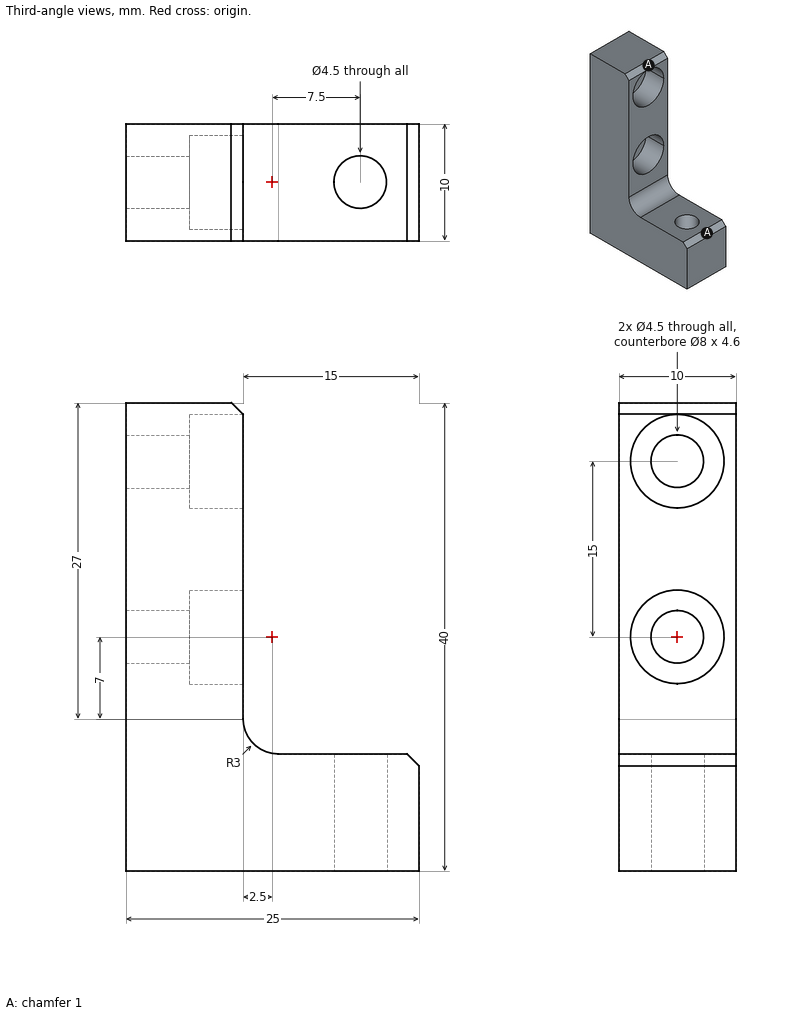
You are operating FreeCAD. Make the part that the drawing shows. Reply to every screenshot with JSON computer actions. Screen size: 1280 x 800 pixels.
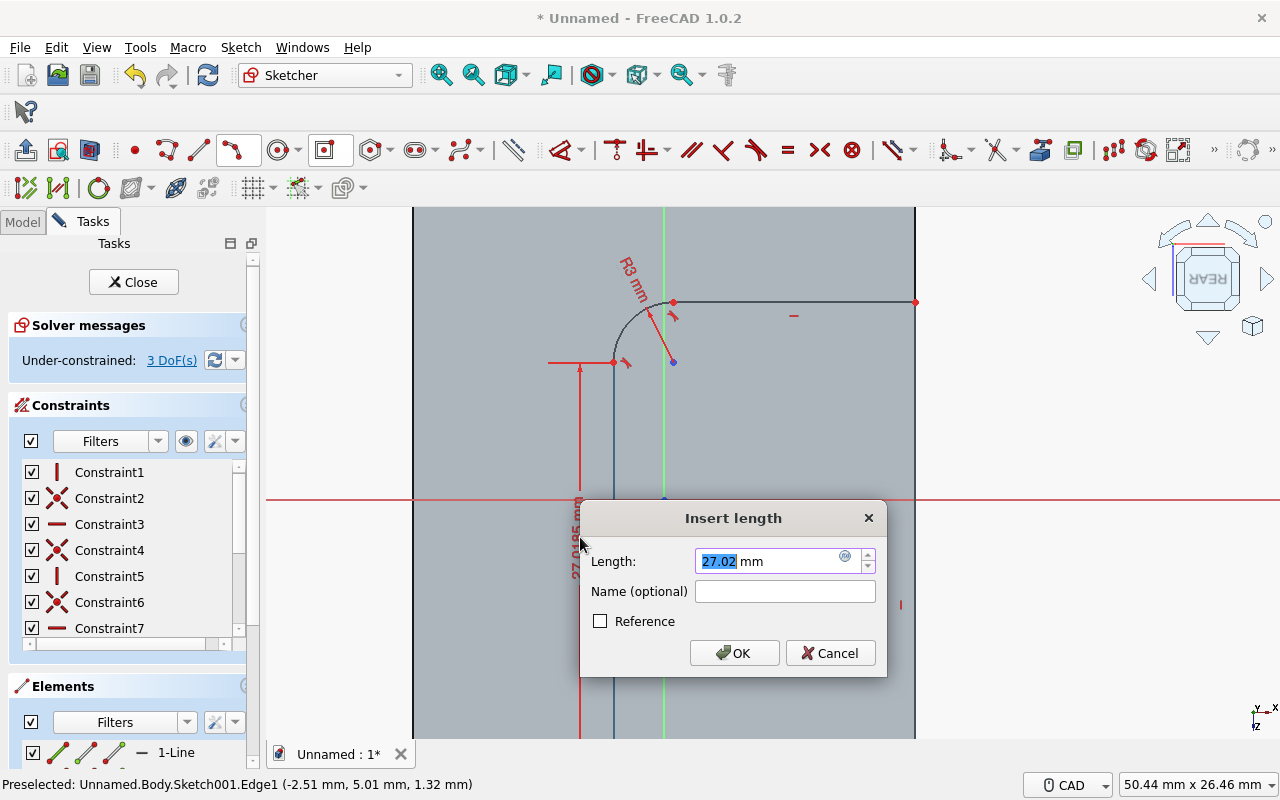
{"action": "type", "text": "27"}
{"action": "key", "text": "Return"}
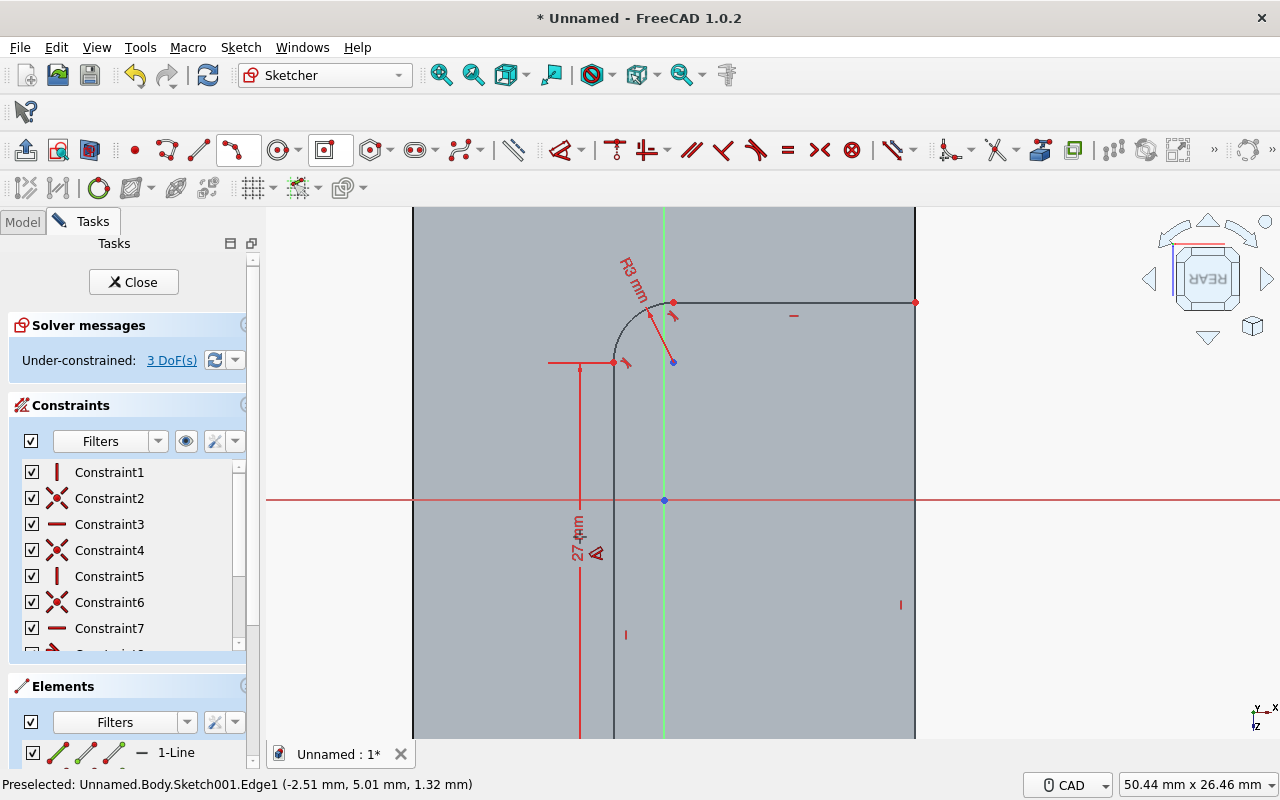
{"action": "scroll", "coordinate": [631, 317], "scroll_direction": "down", "scroll_amount": 3}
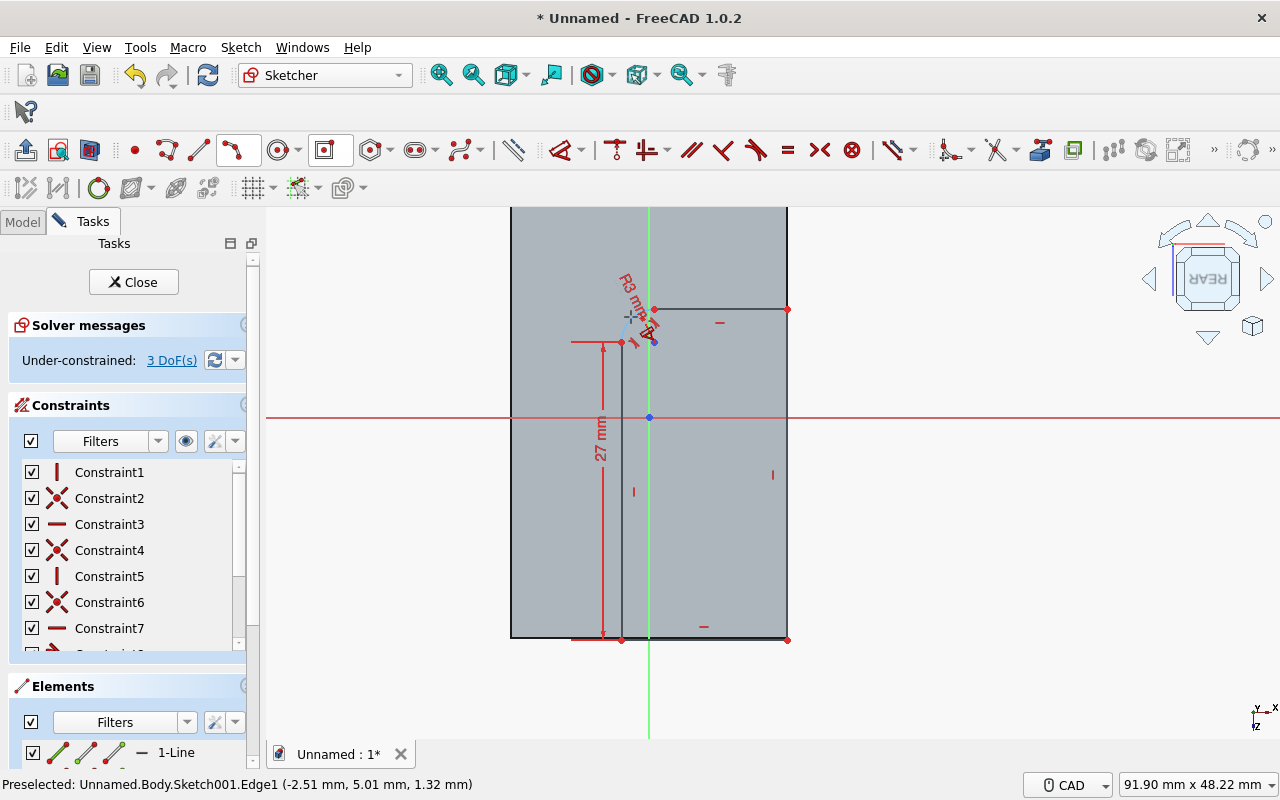
{"action": "left_click", "coordinate": [671, 640]}
{"action": "left_click", "coordinate": [704, 674]}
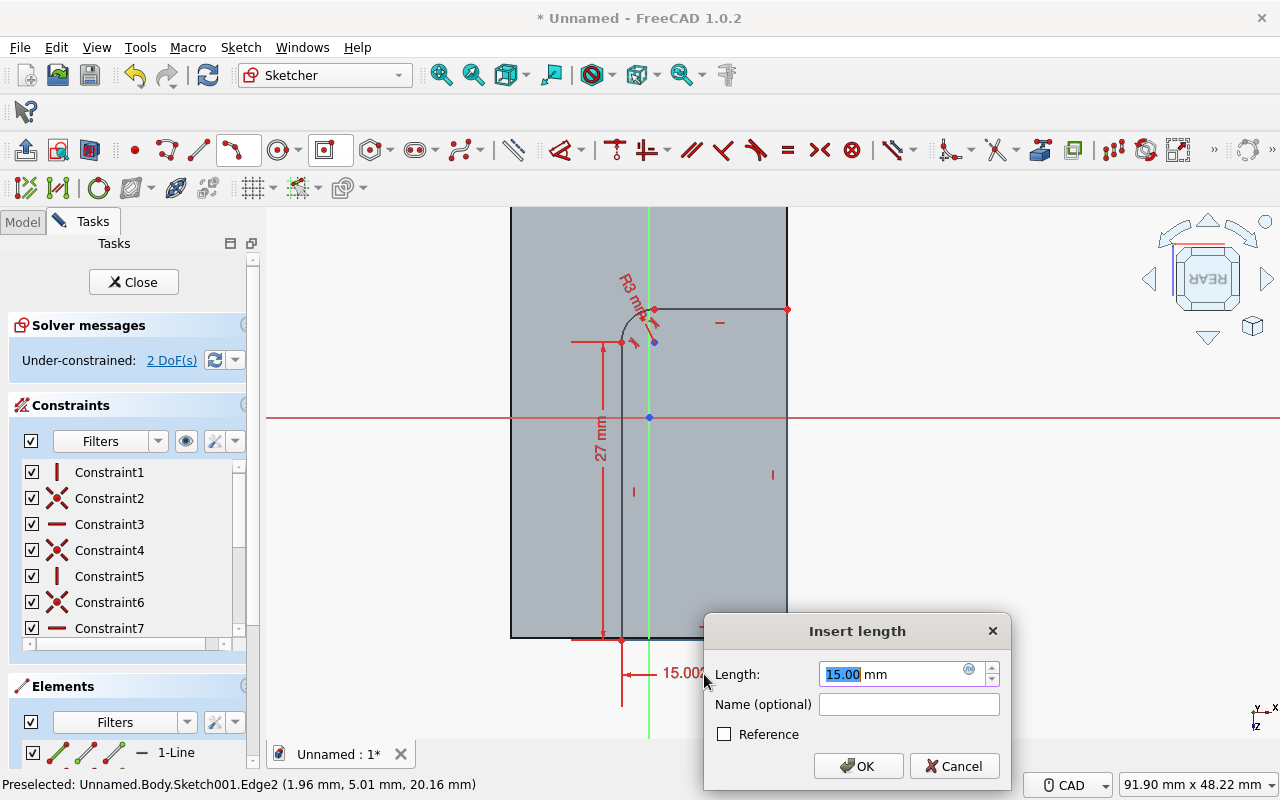
{"action": "type", "text": "15"}
{"action": "key", "text": "Return"}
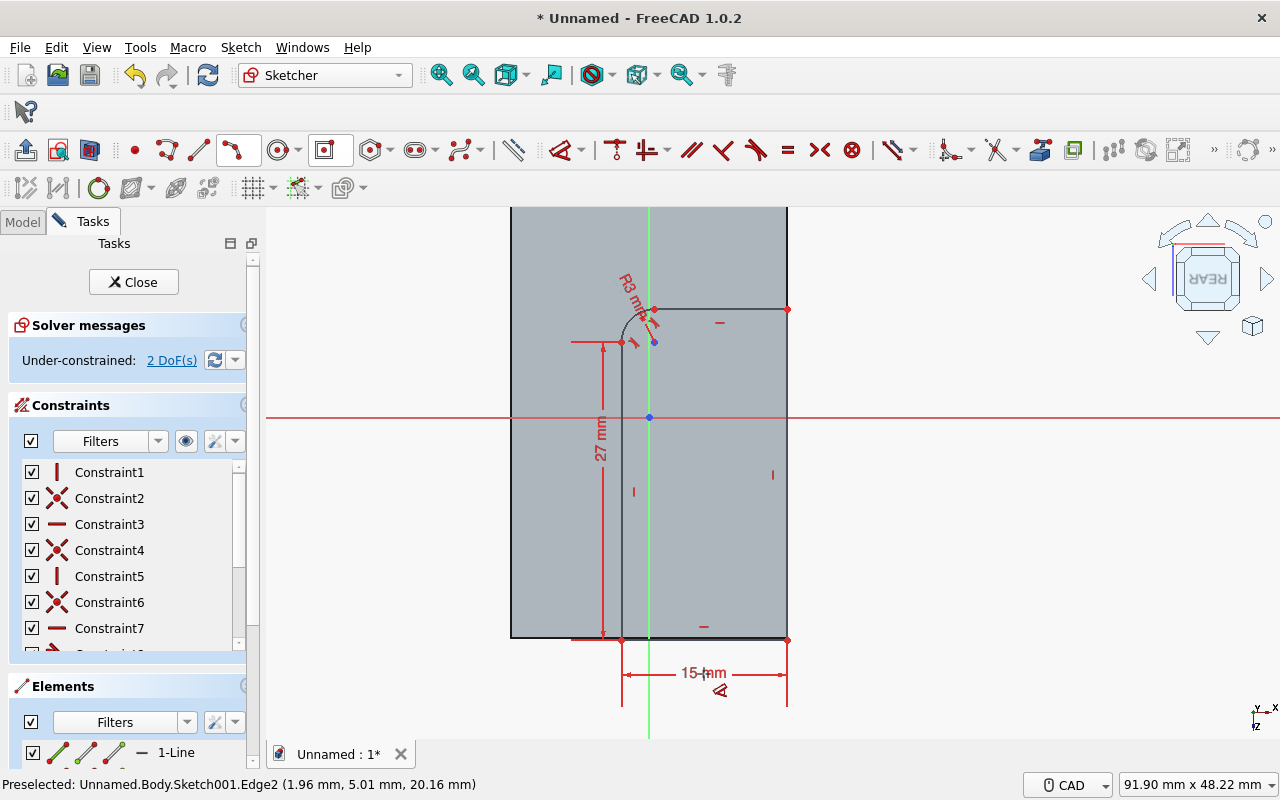
{"action": "left_click", "coordinate": [622, 342]}
{"action": "left_click", "coordinate": [588, 380]}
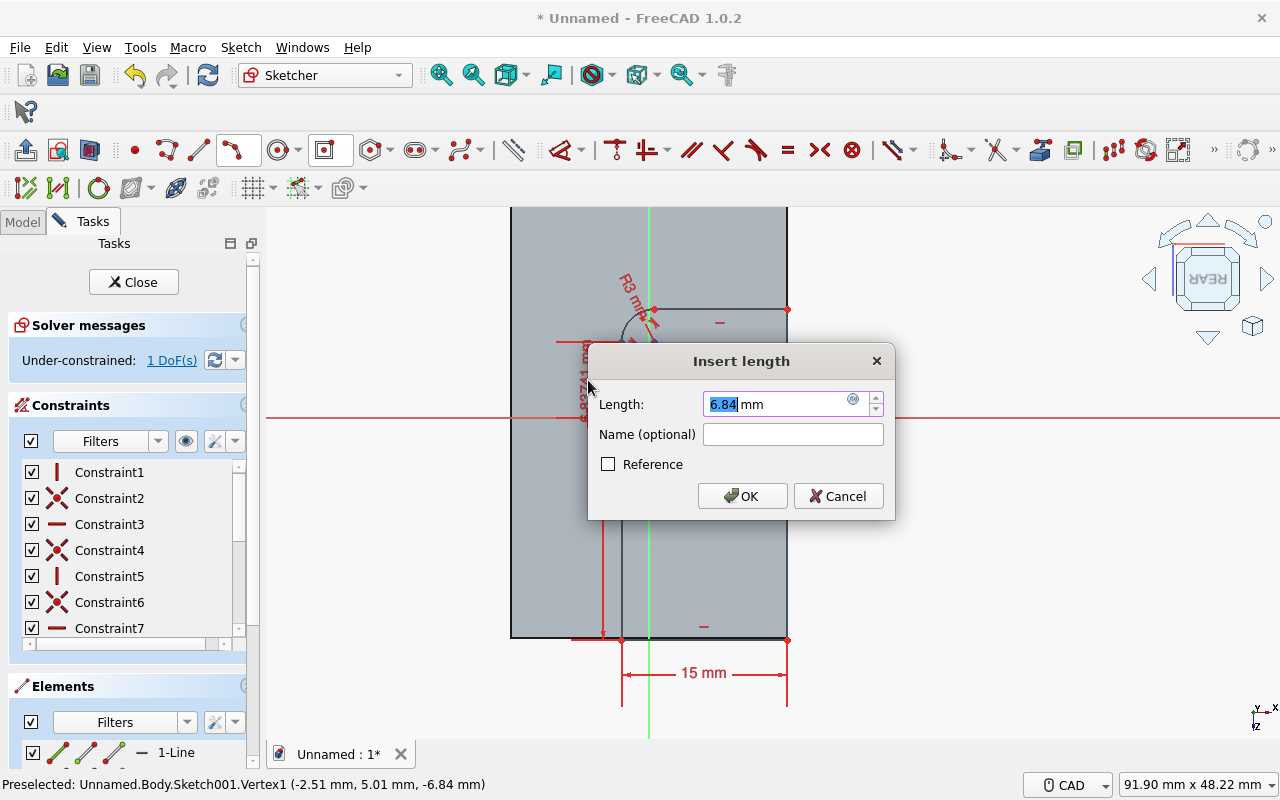
{"action": "type", "text": "7"}
{"action": "key", "text": "Return"}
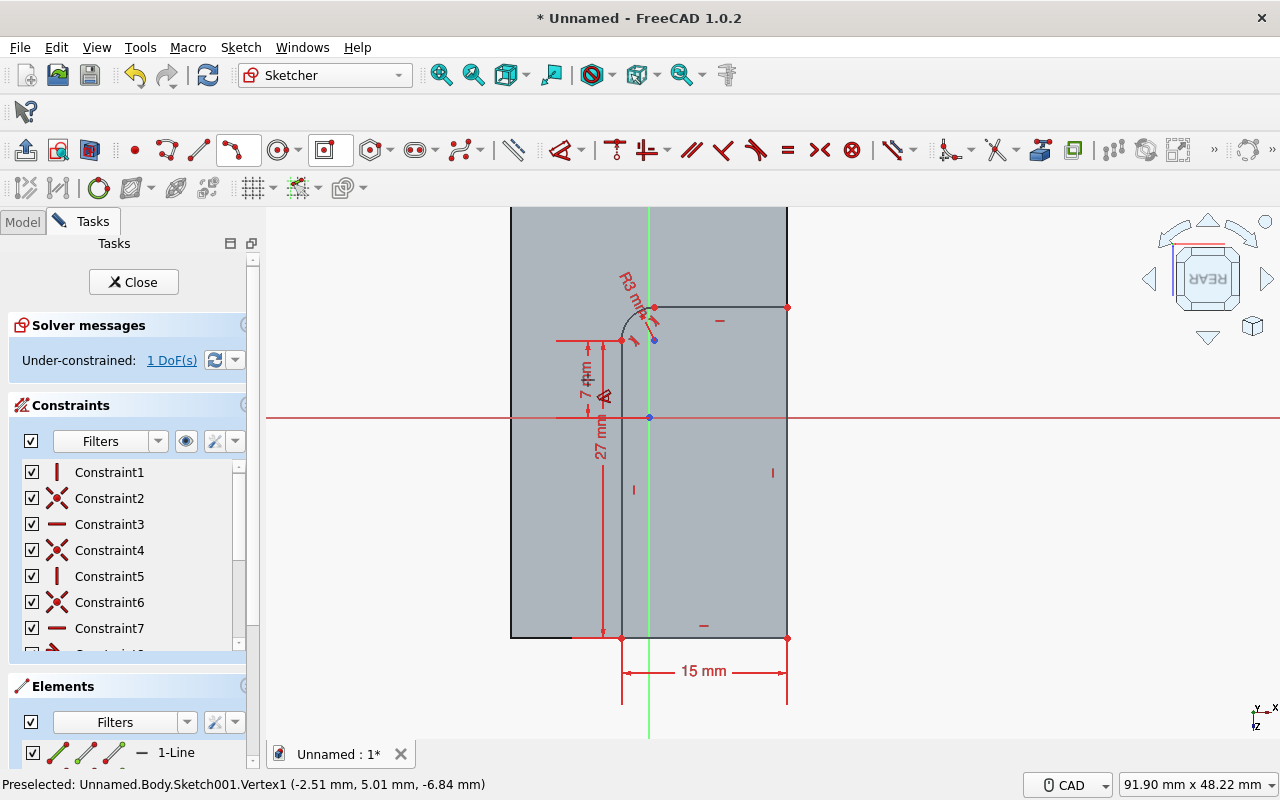
{"action": "scroll", "coordinate": [622, 341], "scroll_direction": "up", "scroll_amount": 2}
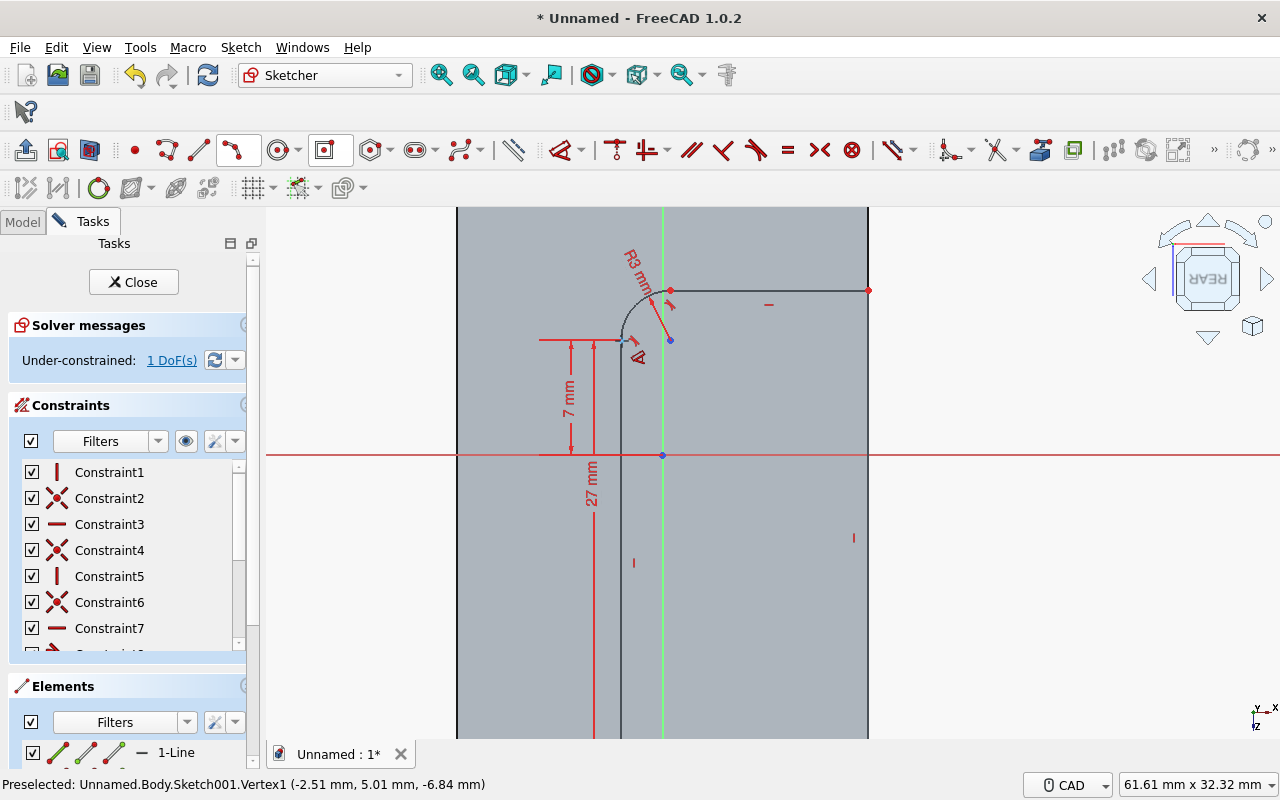
{"action": "left_click", "coordinate": [621, 340]}
{"action": "left_click", "coordinate": [642, 513]}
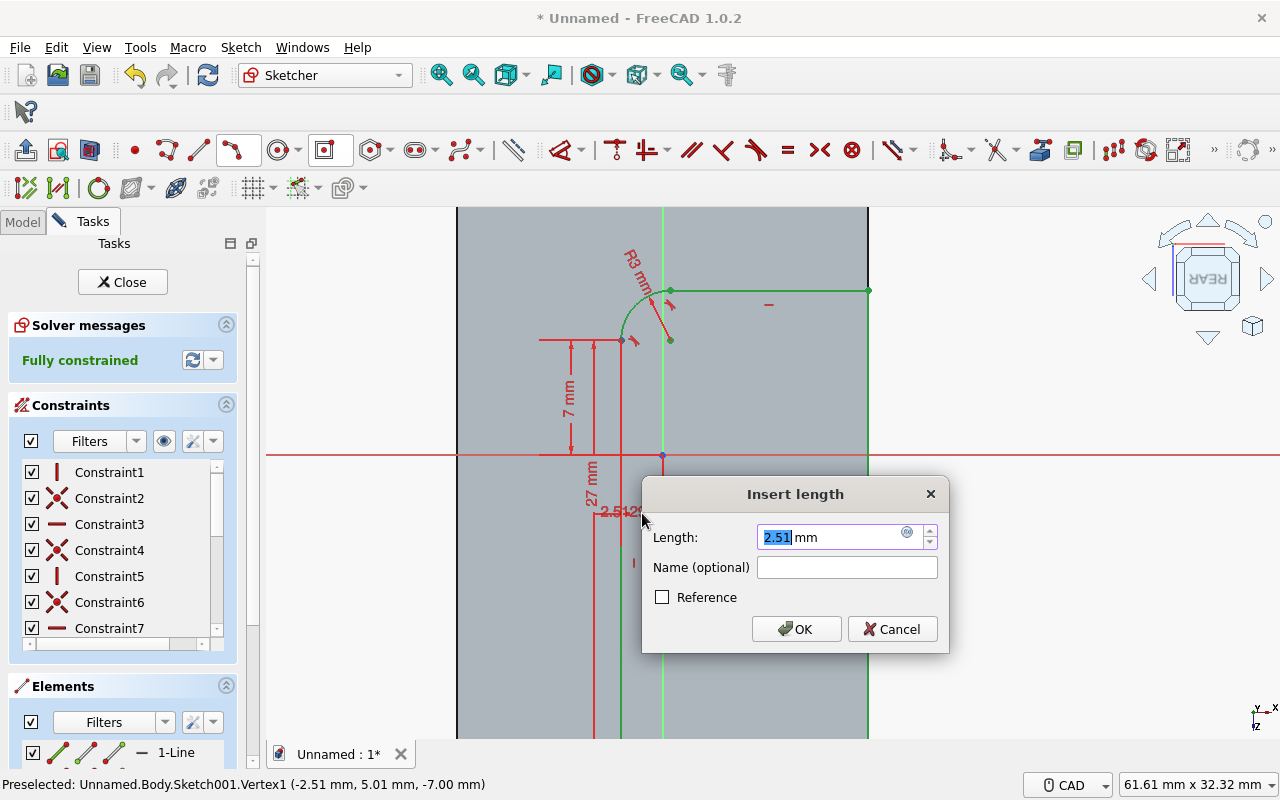
{"action": "type", "text": "2.5"}
{"action": "key", "text": "Return"}
{"action": "key", "text": "Escape"}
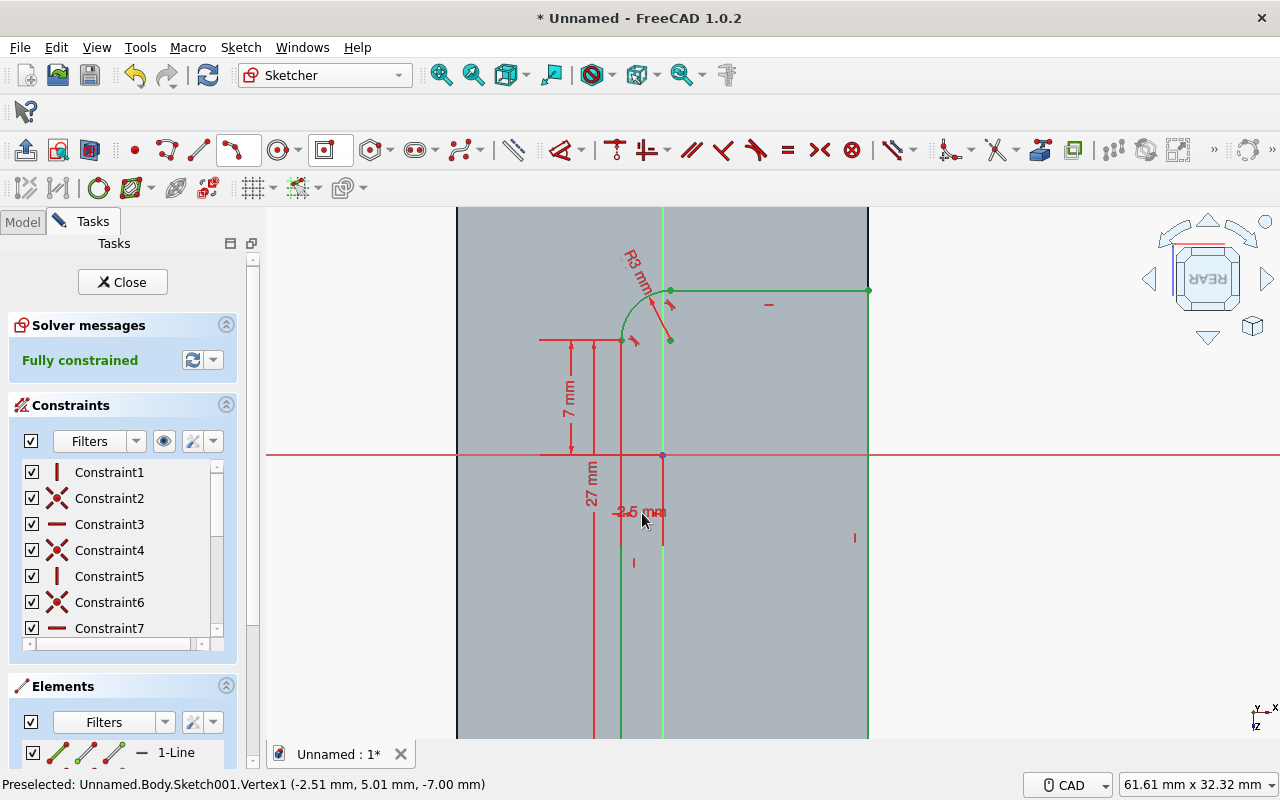
{"action": "left_click", "coordinate": [123, 282]}